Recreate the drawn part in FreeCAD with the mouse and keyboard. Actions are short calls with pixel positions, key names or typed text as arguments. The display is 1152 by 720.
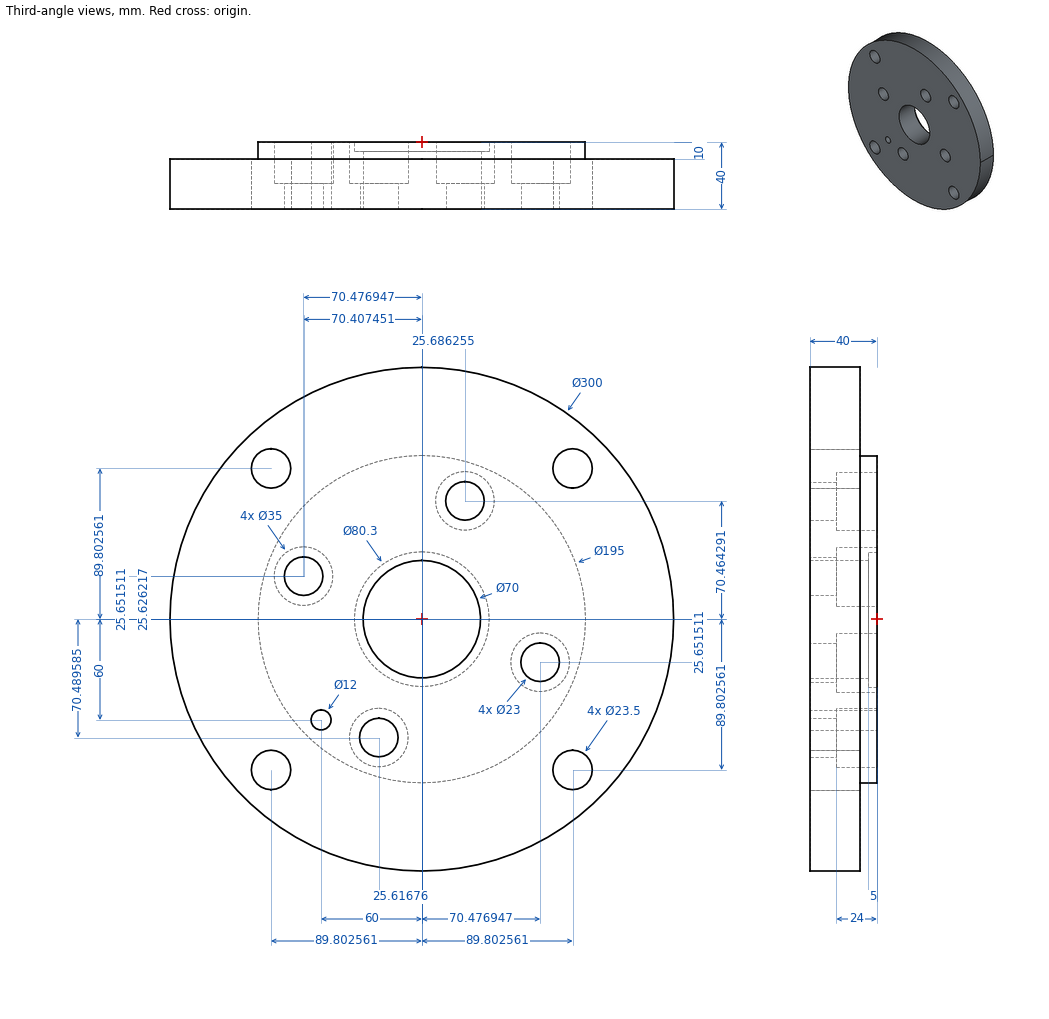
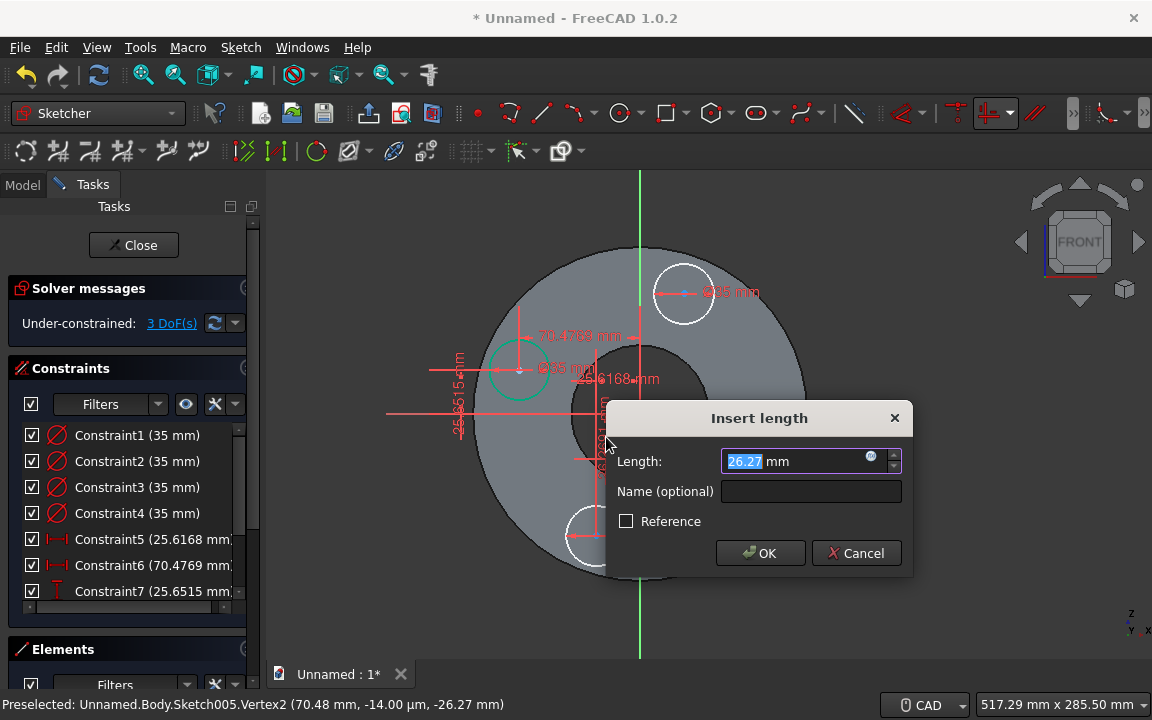
text(25.651511)
key(Return)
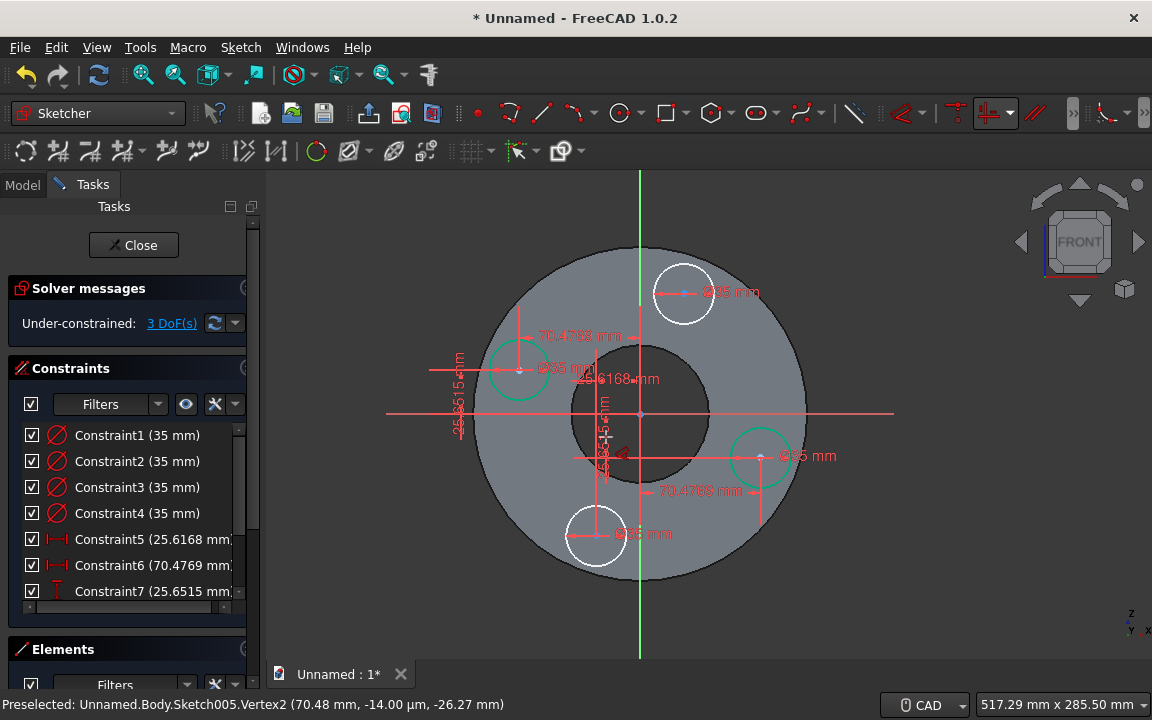
click(596, 536)
click(562, 475)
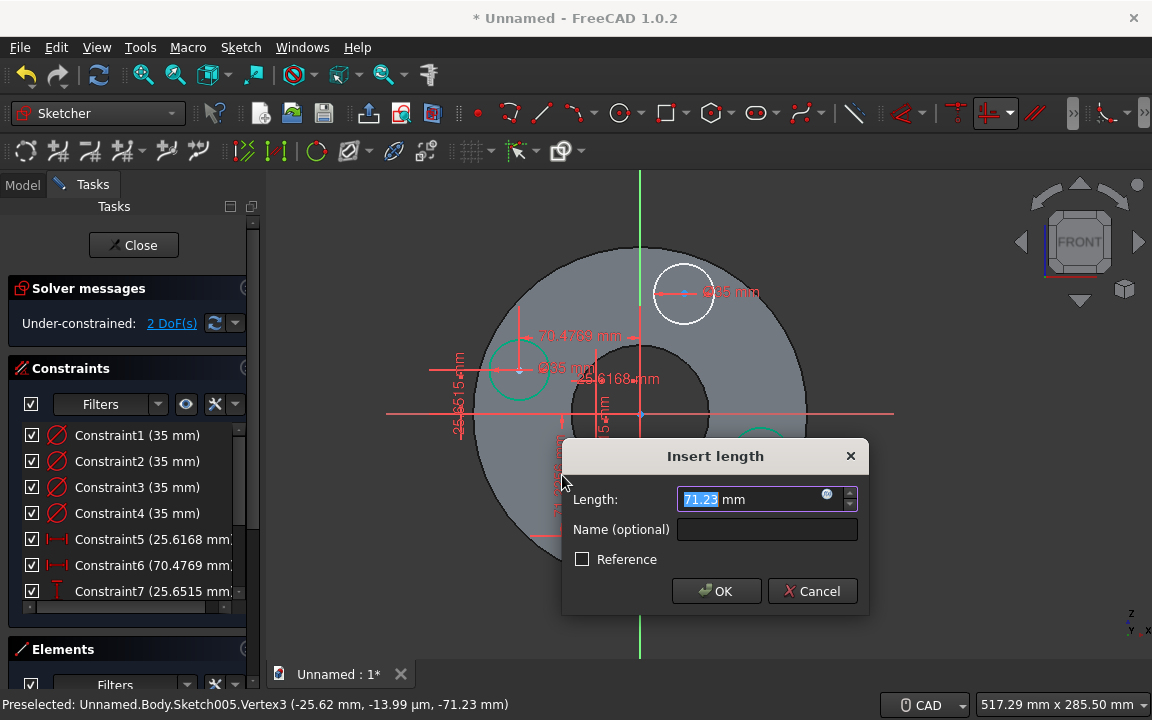
text(70.489585)
key(Return)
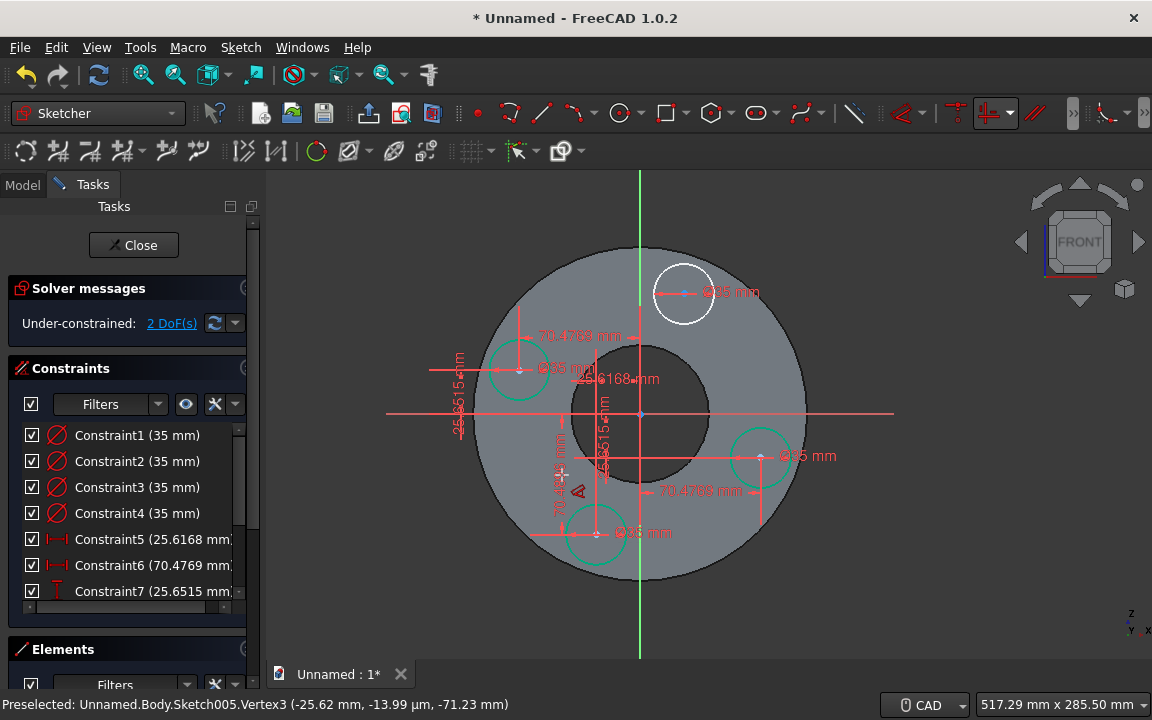
click(684, 294)
click(677, 448)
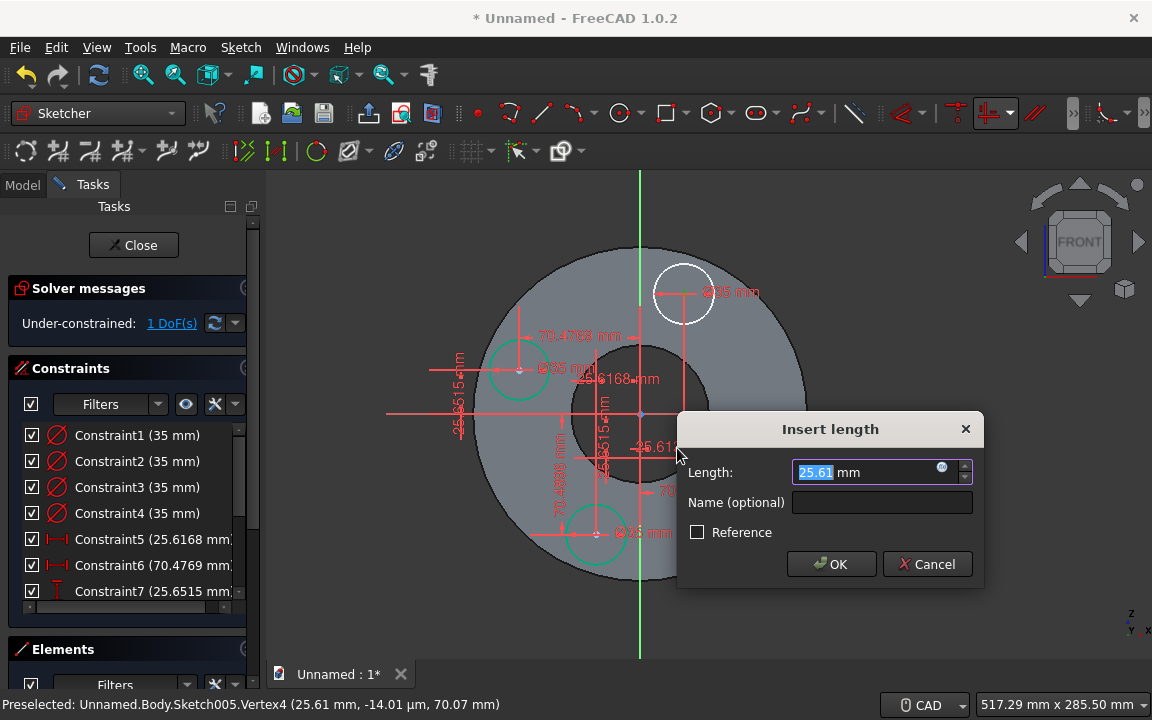
text(25.686255)
key(Return)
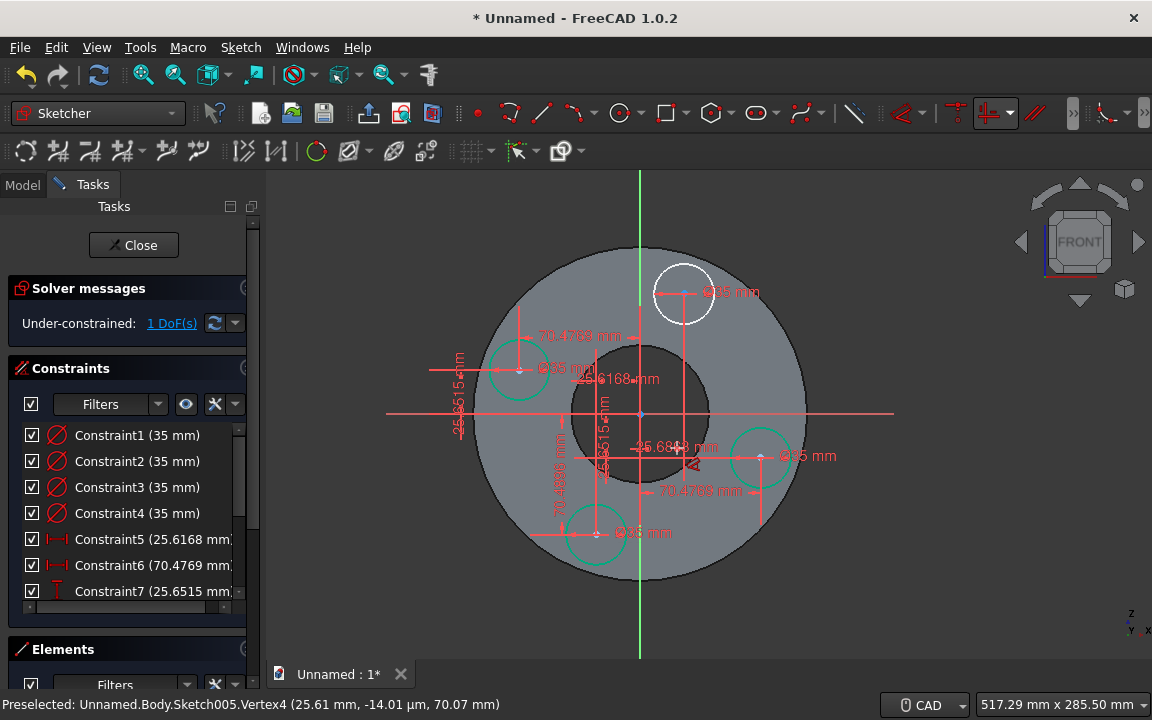
click(684, 294)
click(718, 354)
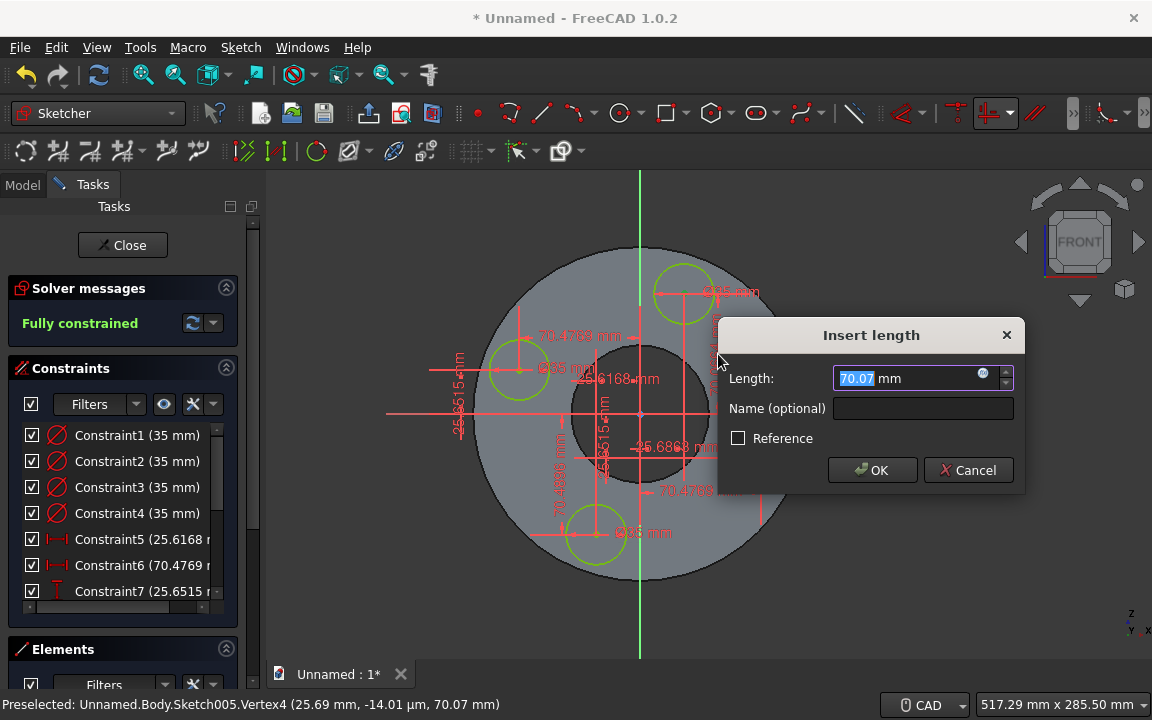
text(70.464291)
key(Return)
key(Escape)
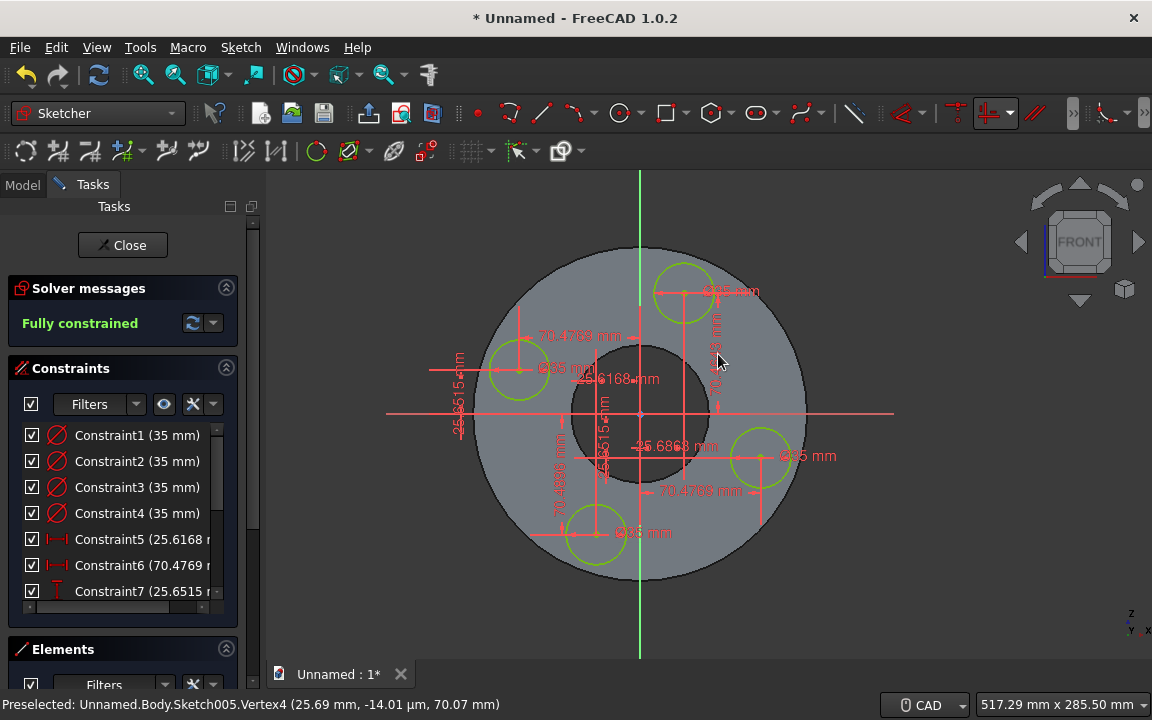
click(123, 245)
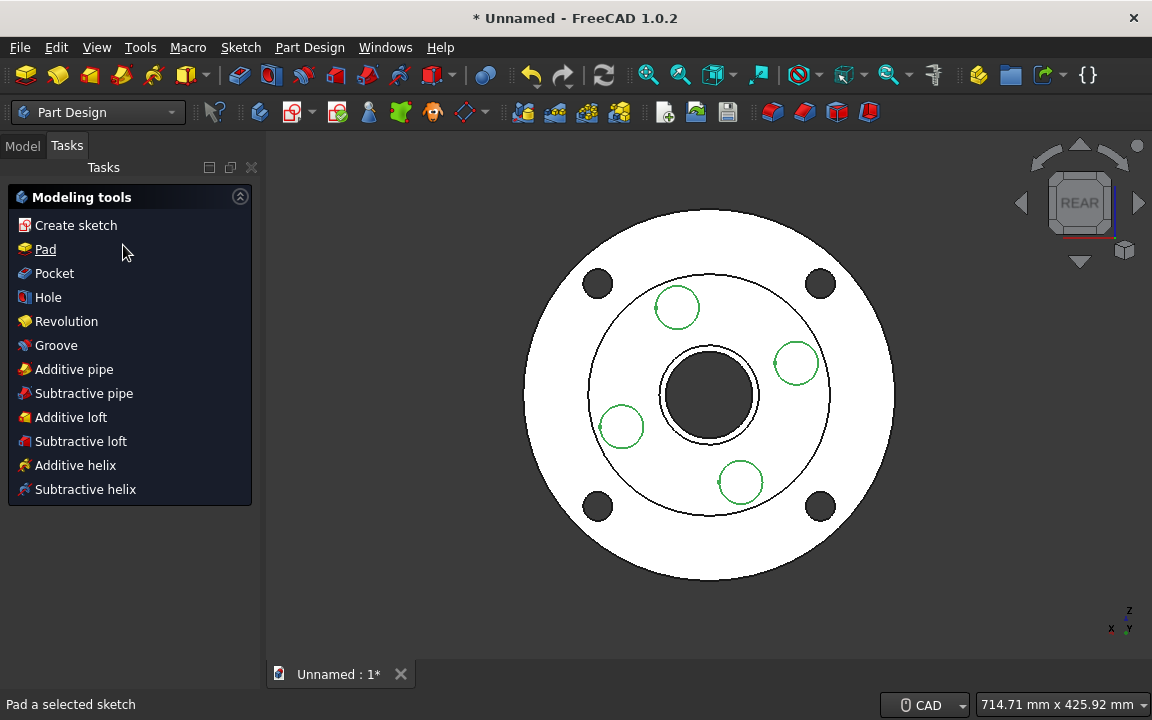
click(240, 76)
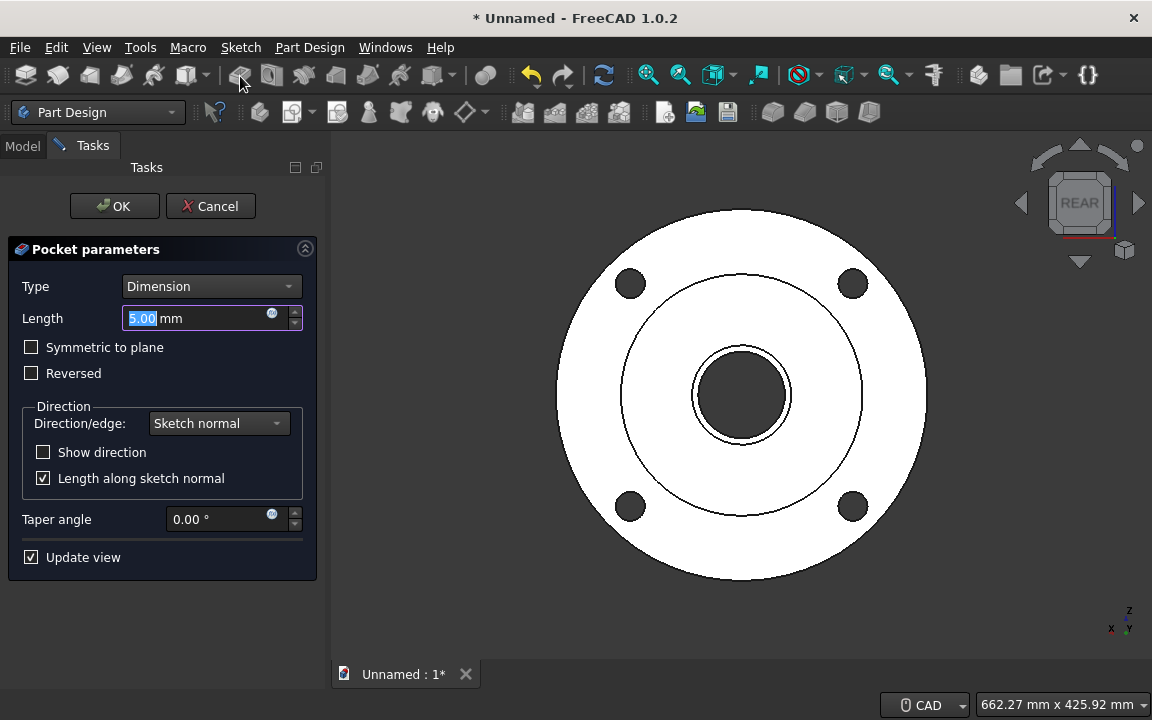
text(24)
key(Tab)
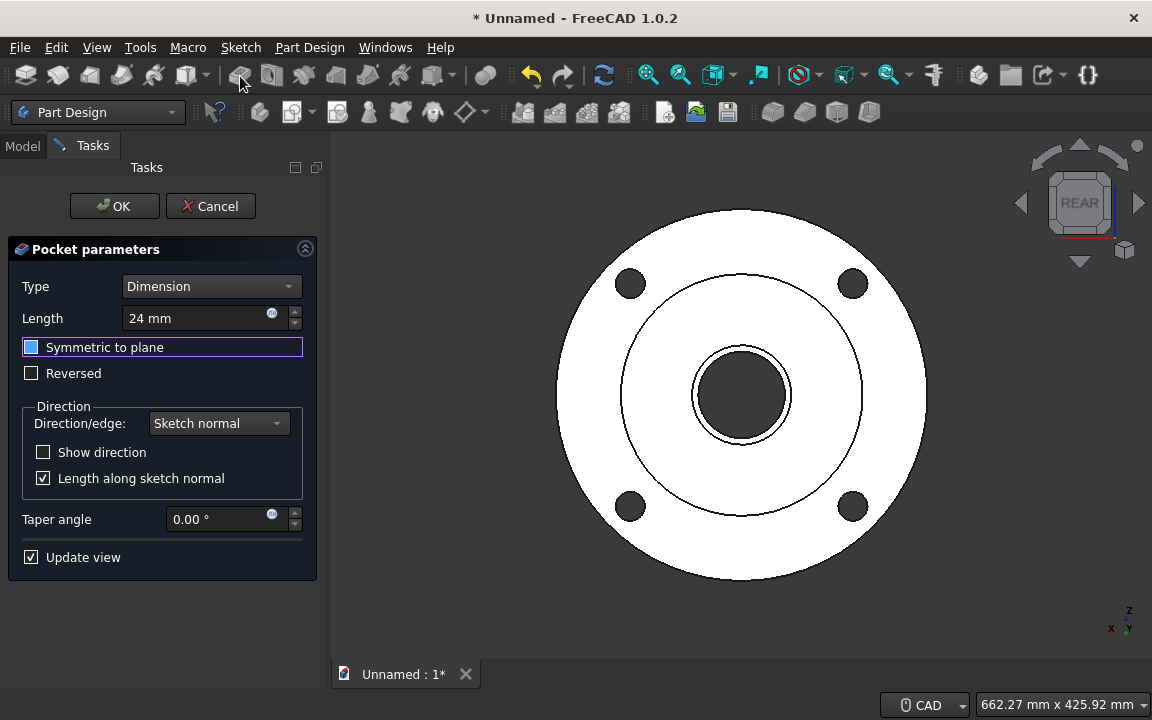
click(30, 373)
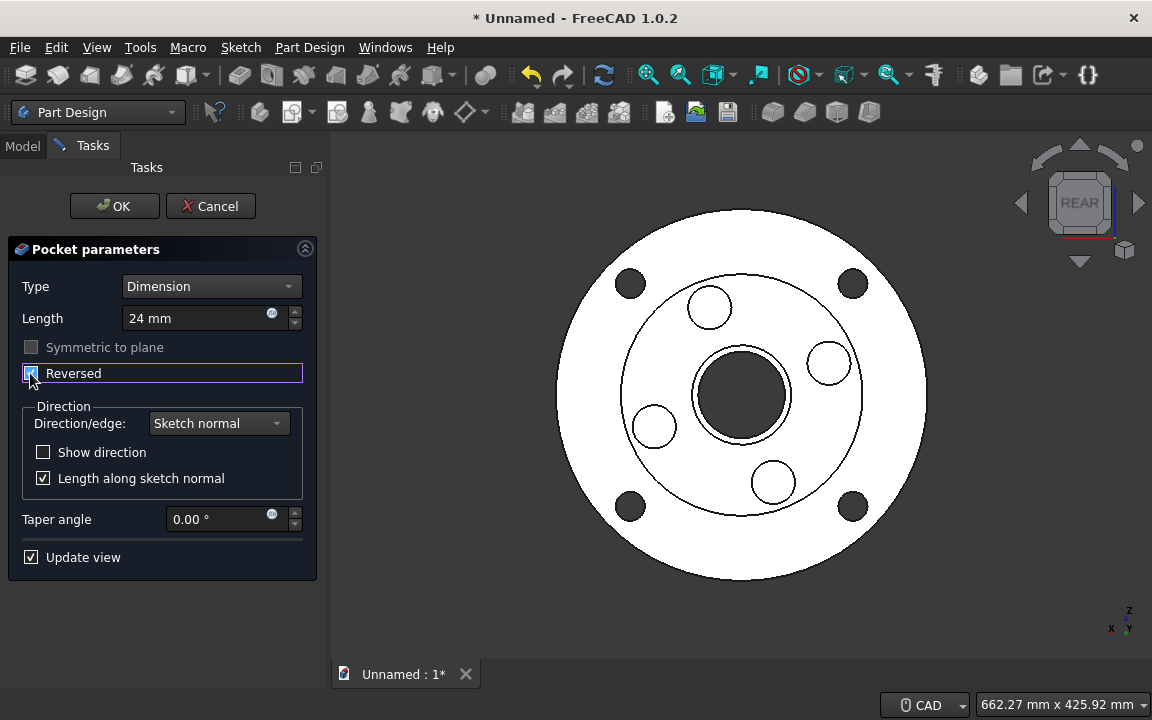
click(115, 206)